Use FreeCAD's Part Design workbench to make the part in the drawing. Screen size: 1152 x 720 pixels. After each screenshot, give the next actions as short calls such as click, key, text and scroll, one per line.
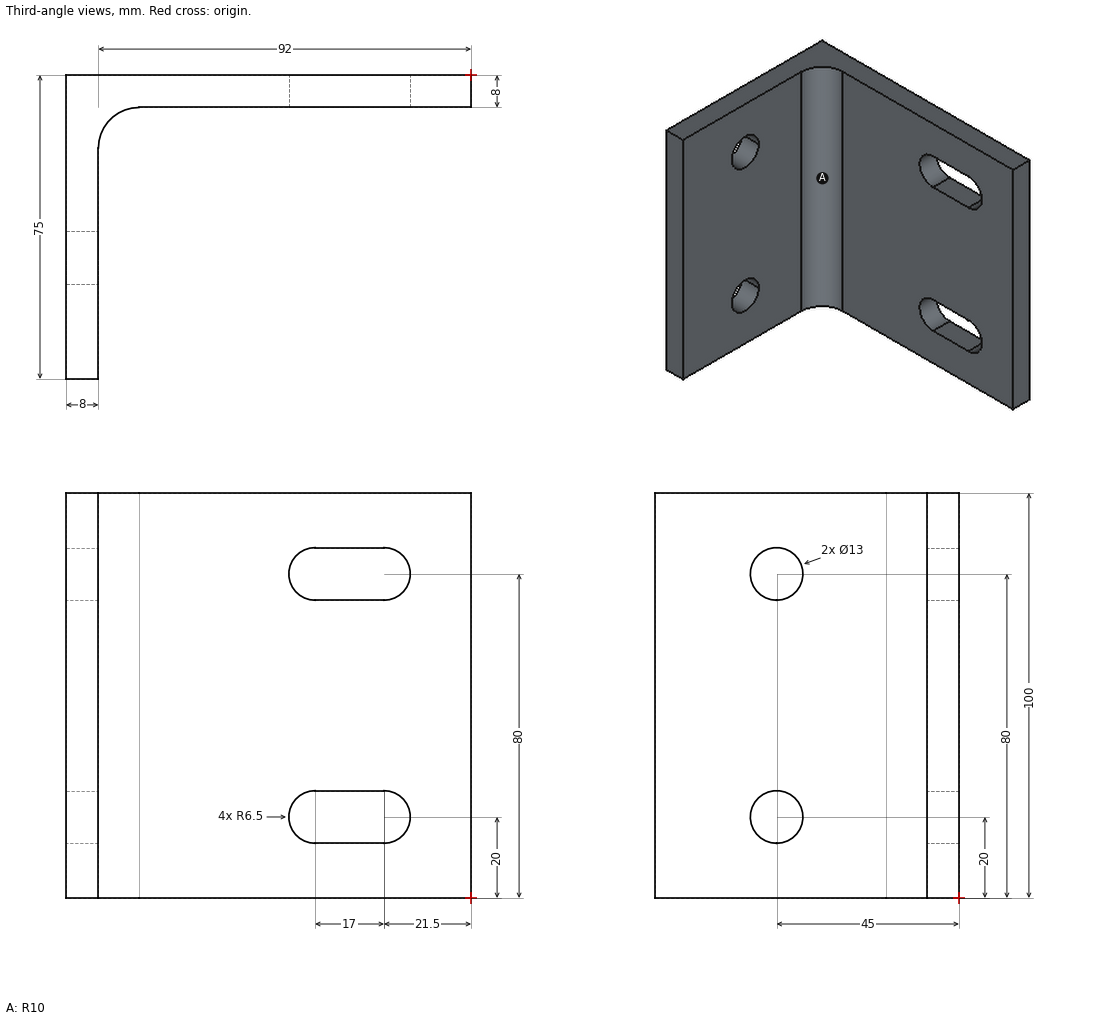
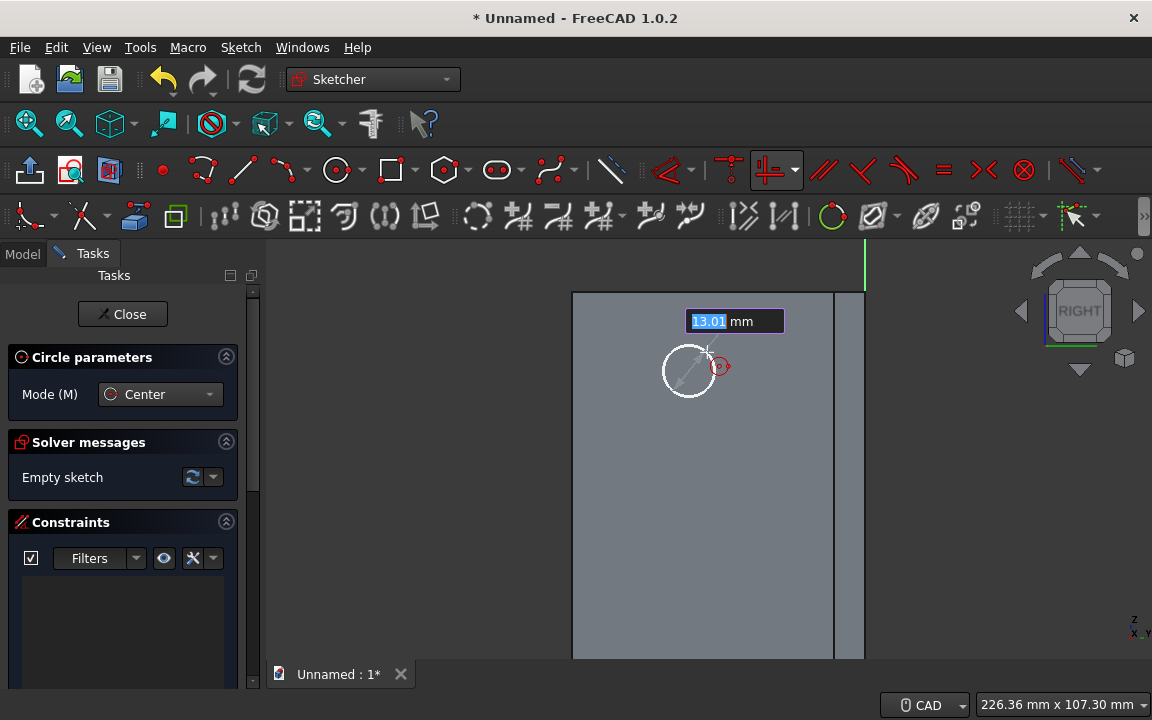
text(13)
key(Return)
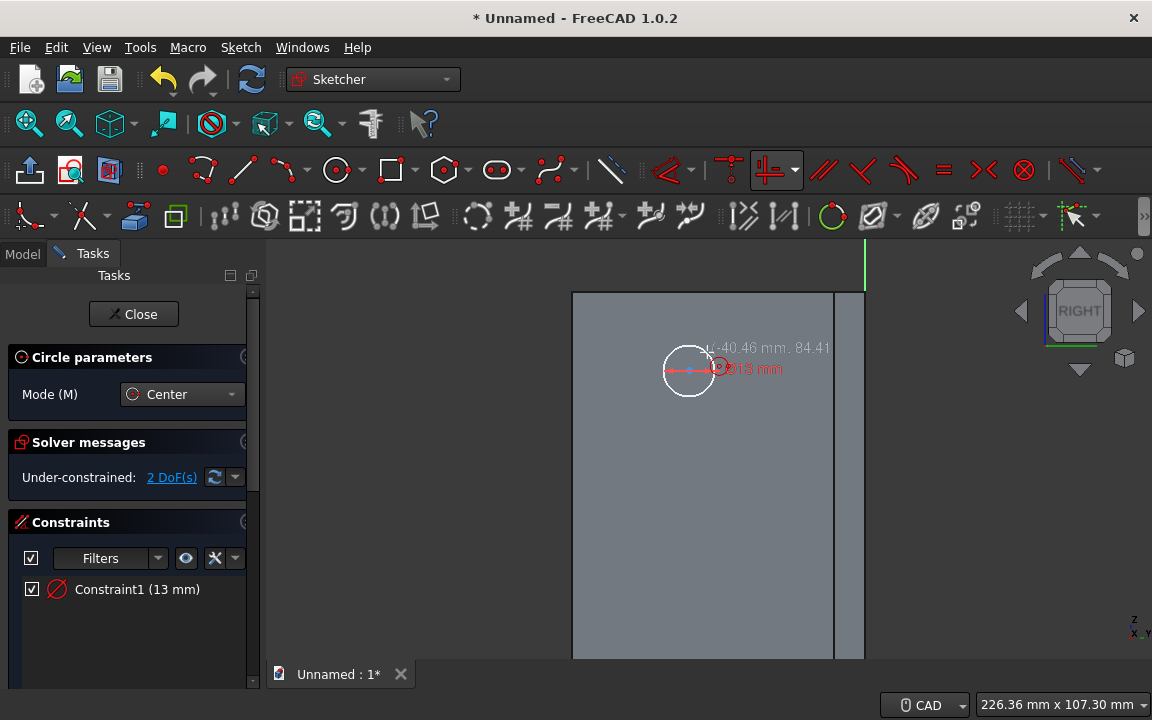
click(689, 605)
move(707, 587)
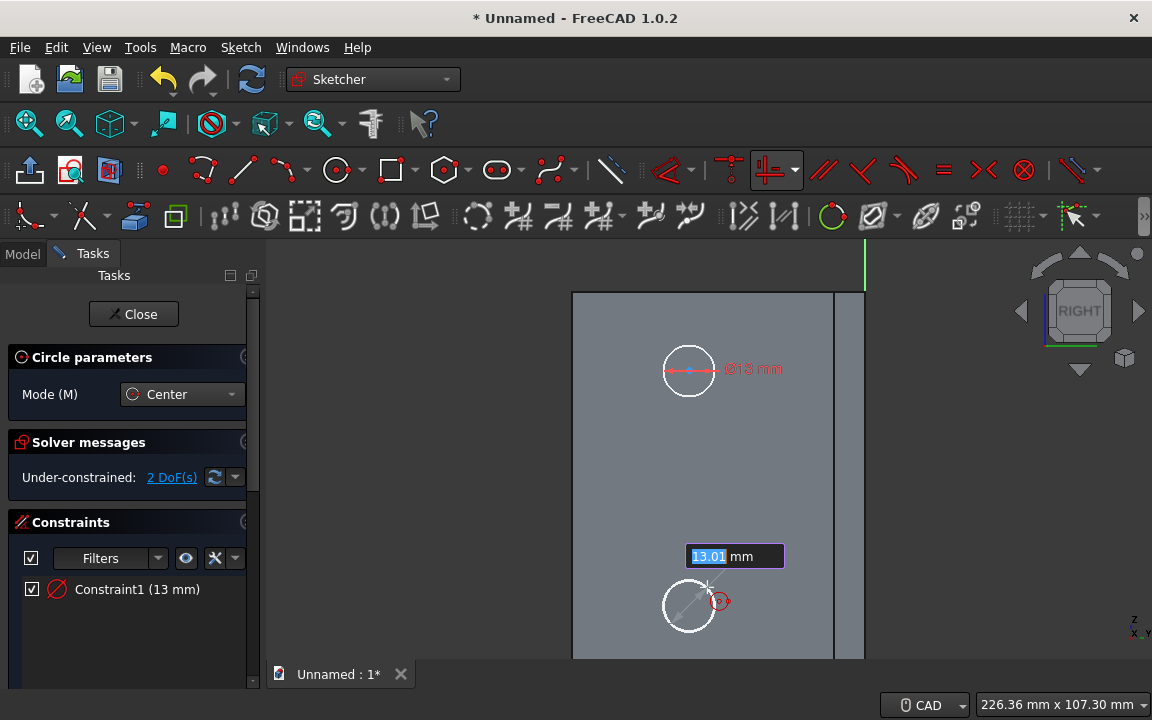
text(13)
key(Return)
key(Escape)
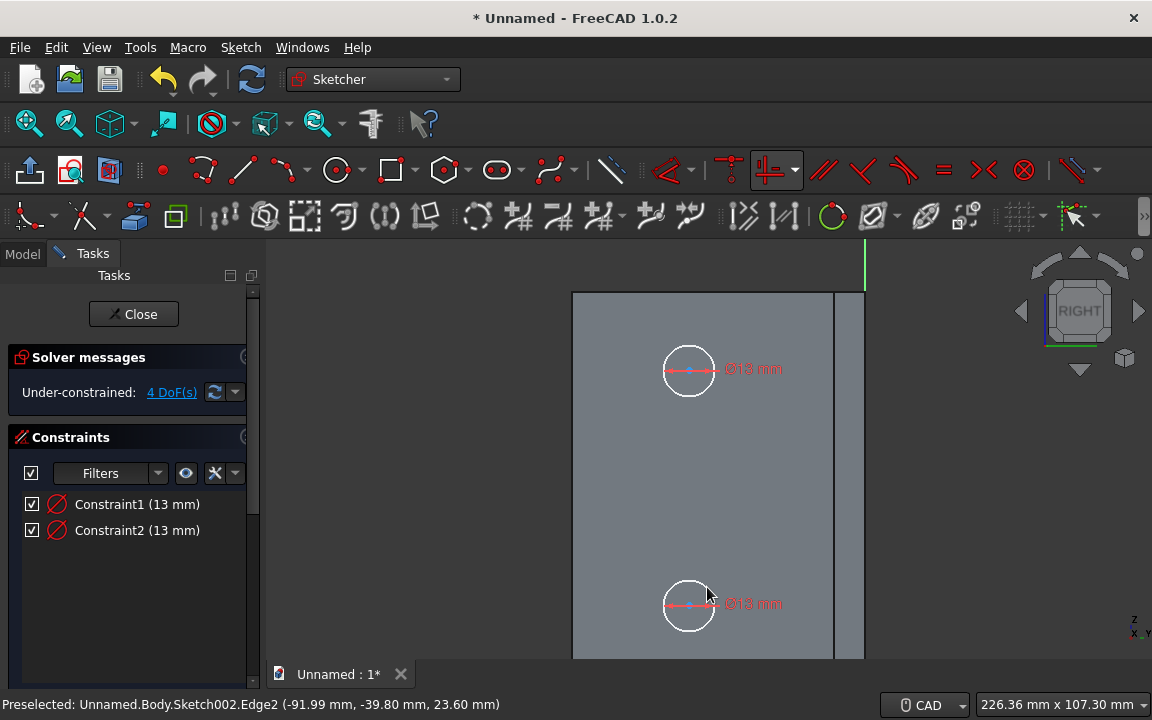
click(666, 170)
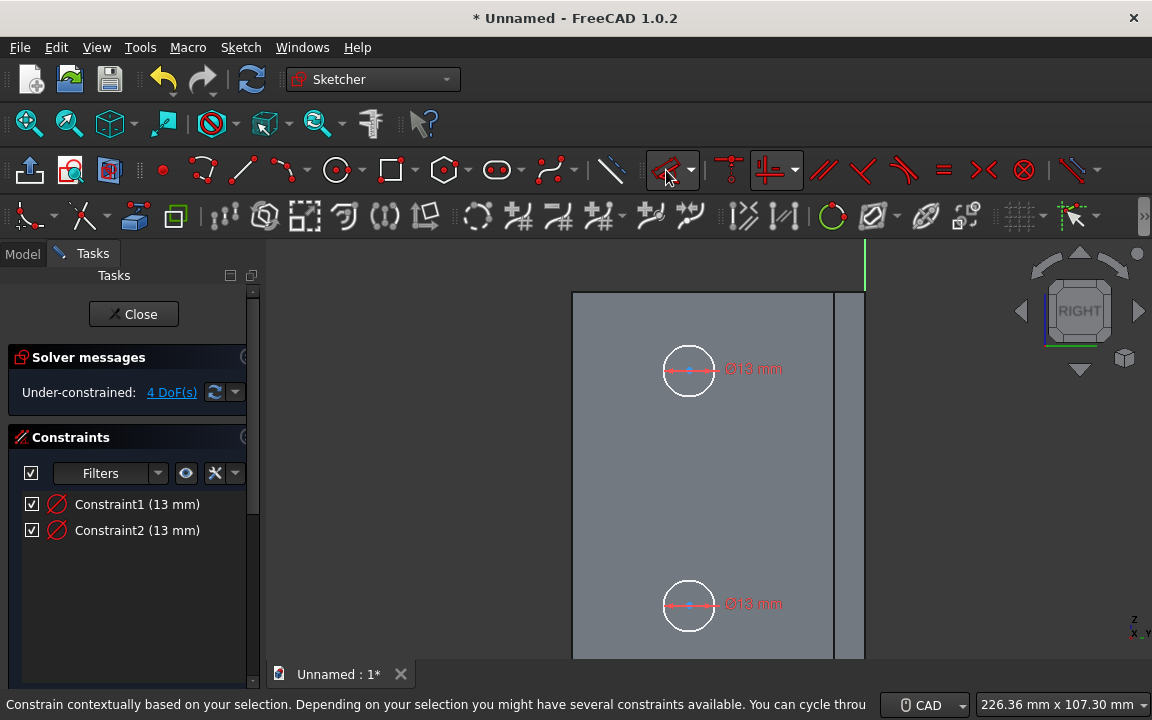
click(689, 371)
click(777, 337)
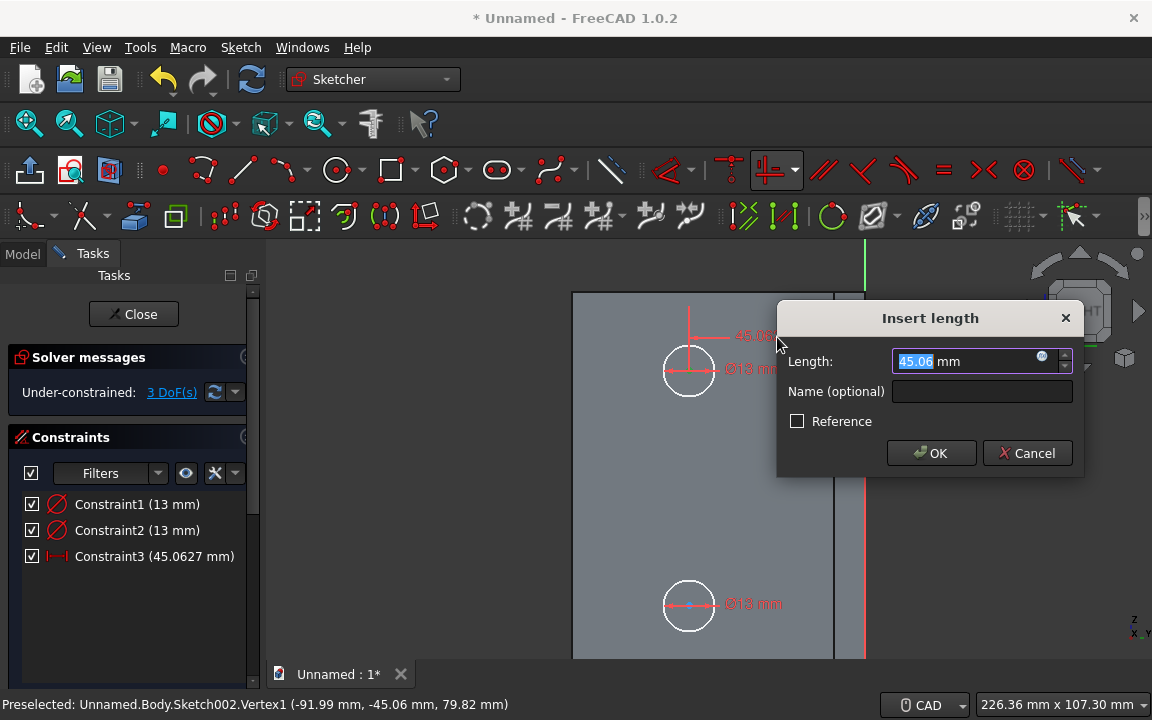
text(45)
key(Return)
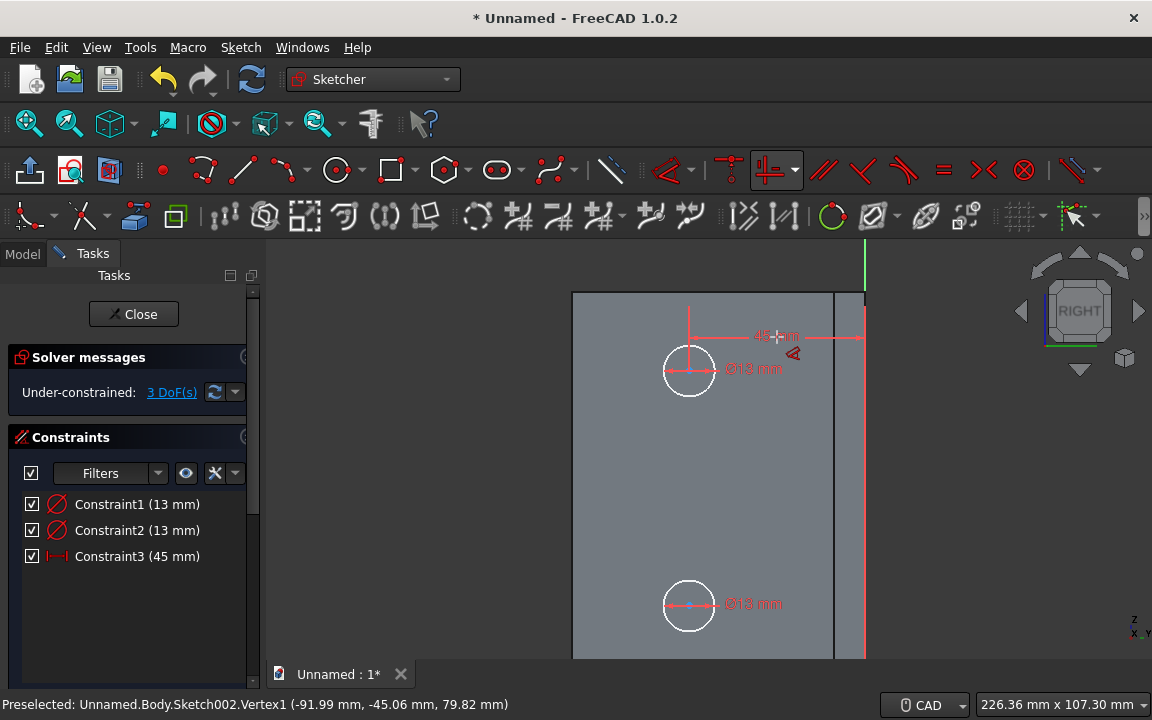
click(689, 371)
click(899, 501)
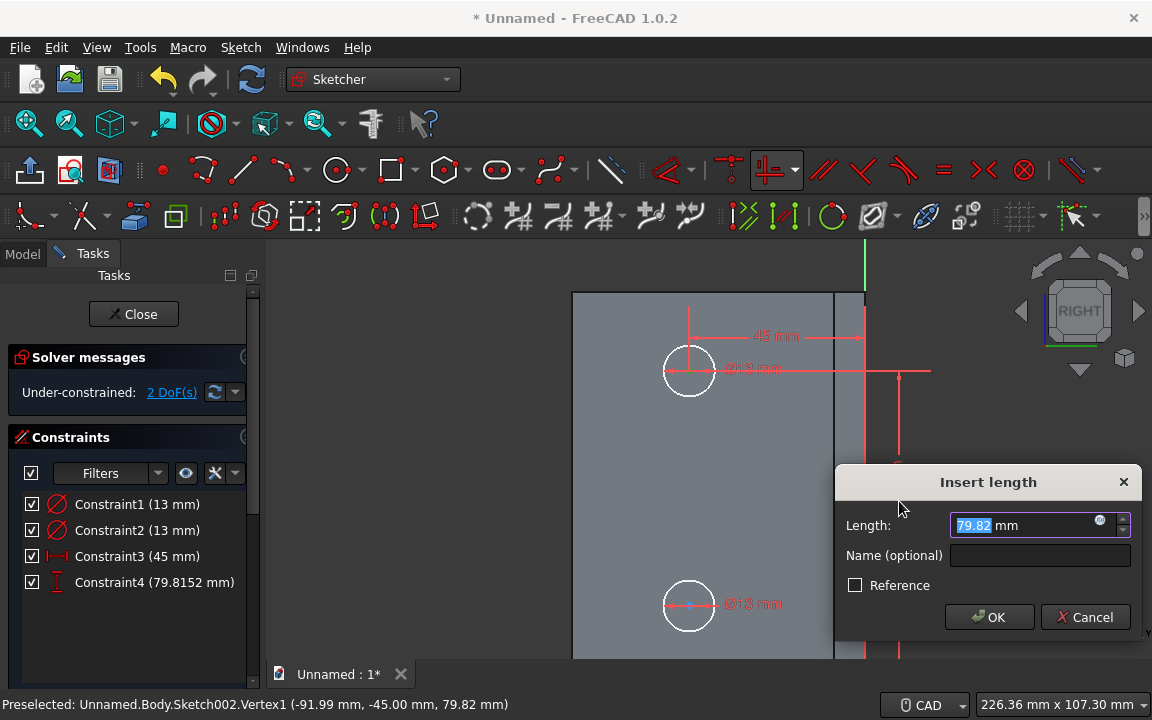
text(80)
key(Return)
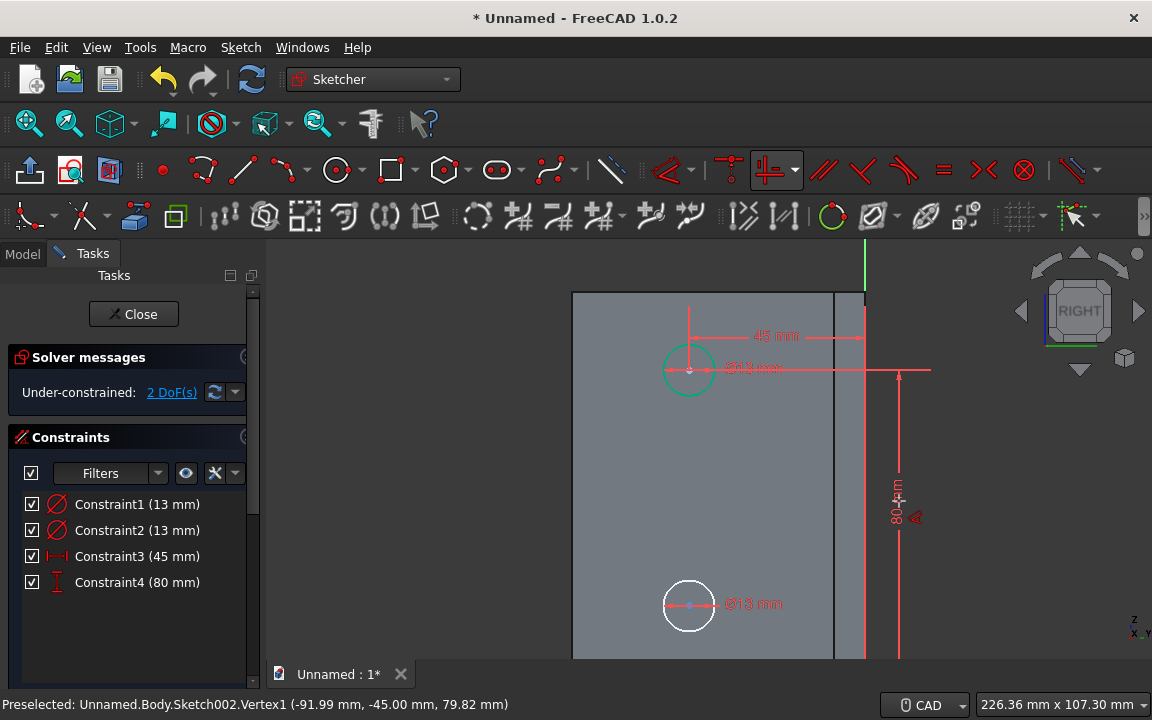
click(689, 606)
click(777, 572)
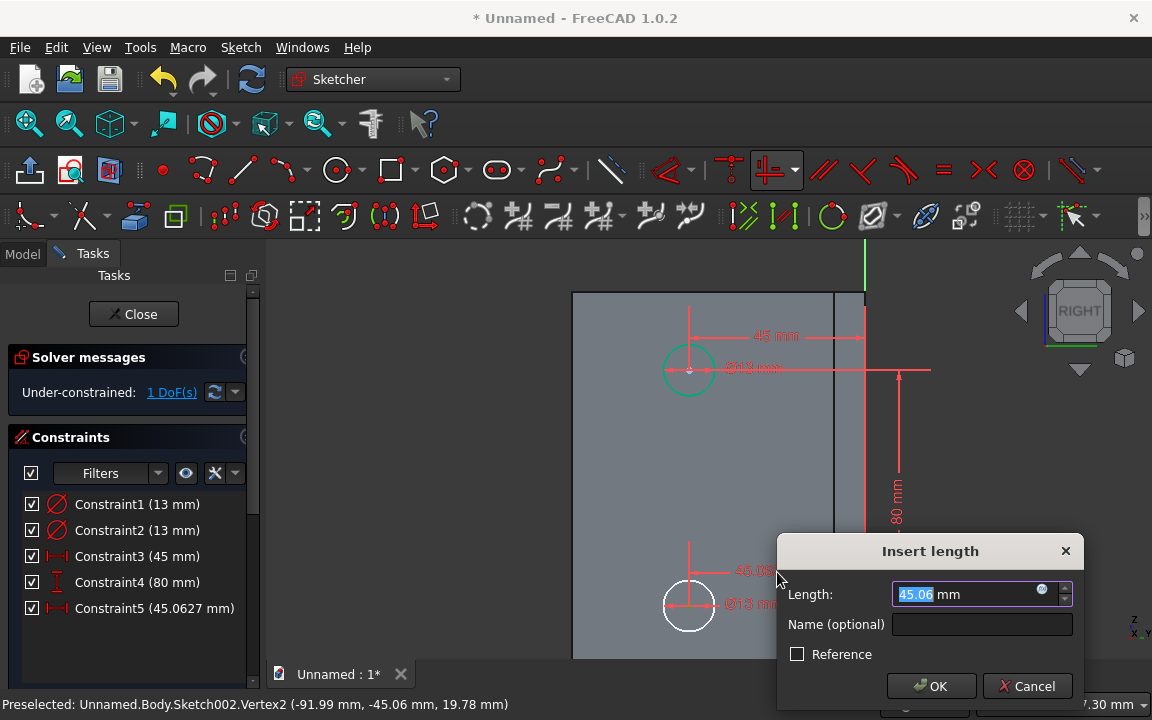
text(45)
key(Return)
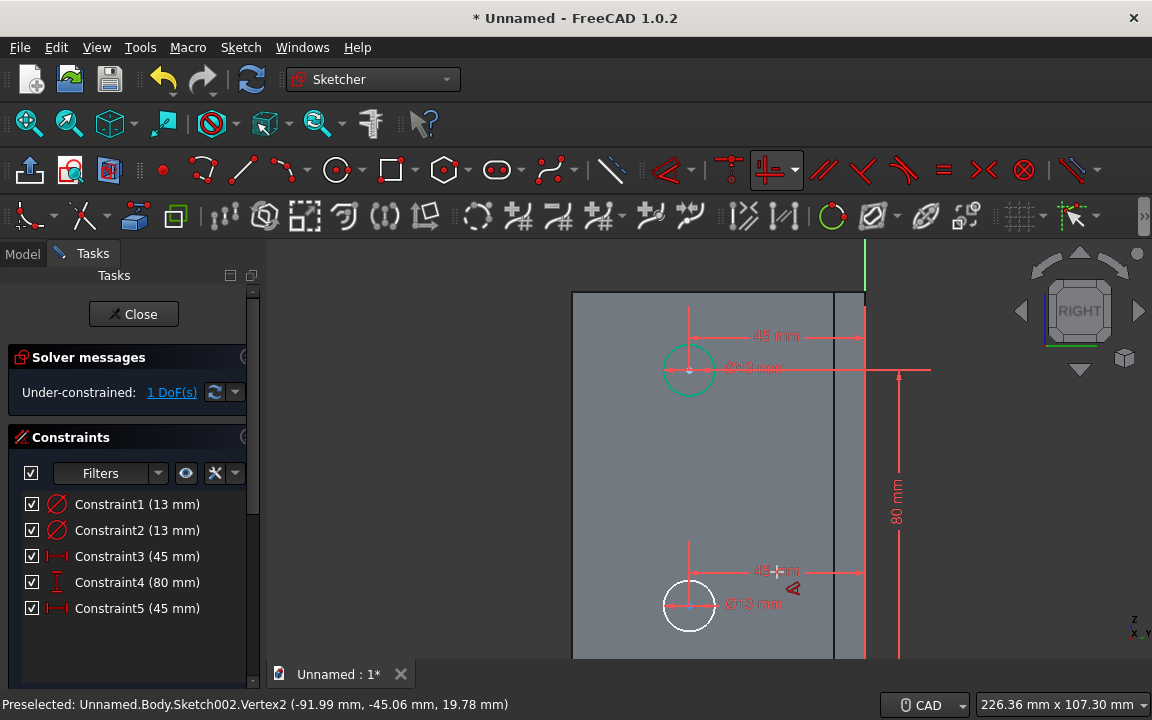
click(689, 606)
click(899, 618)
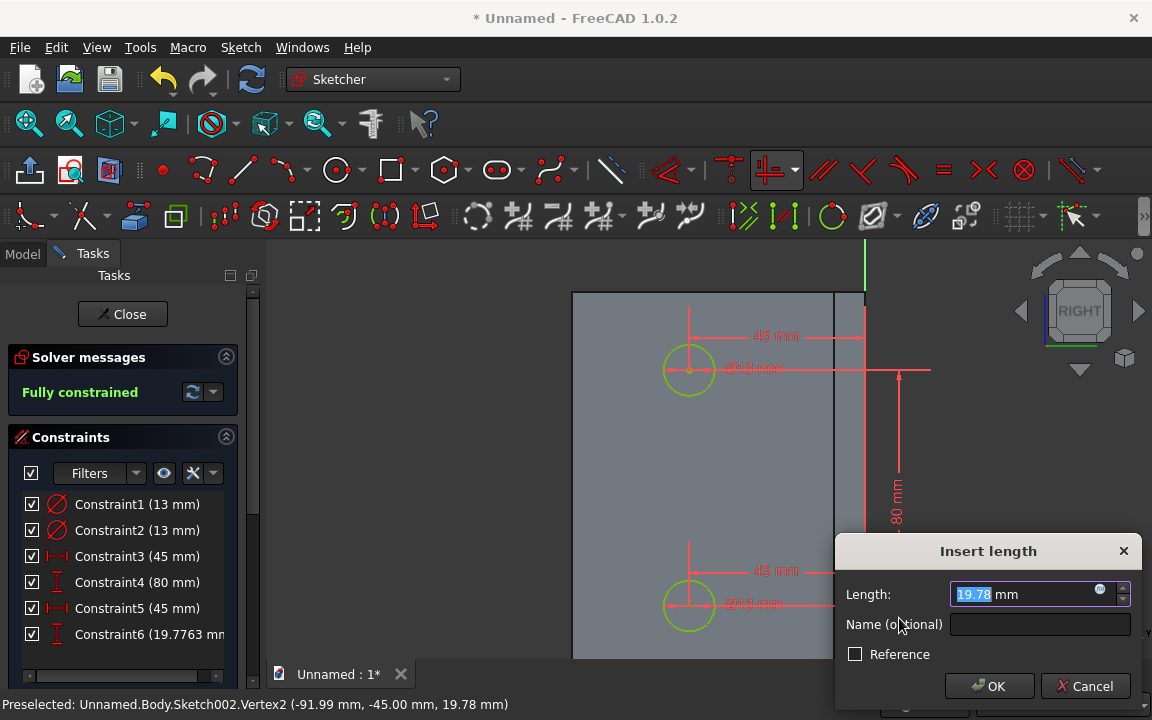
text(20)
key(Return)
key(Escape)